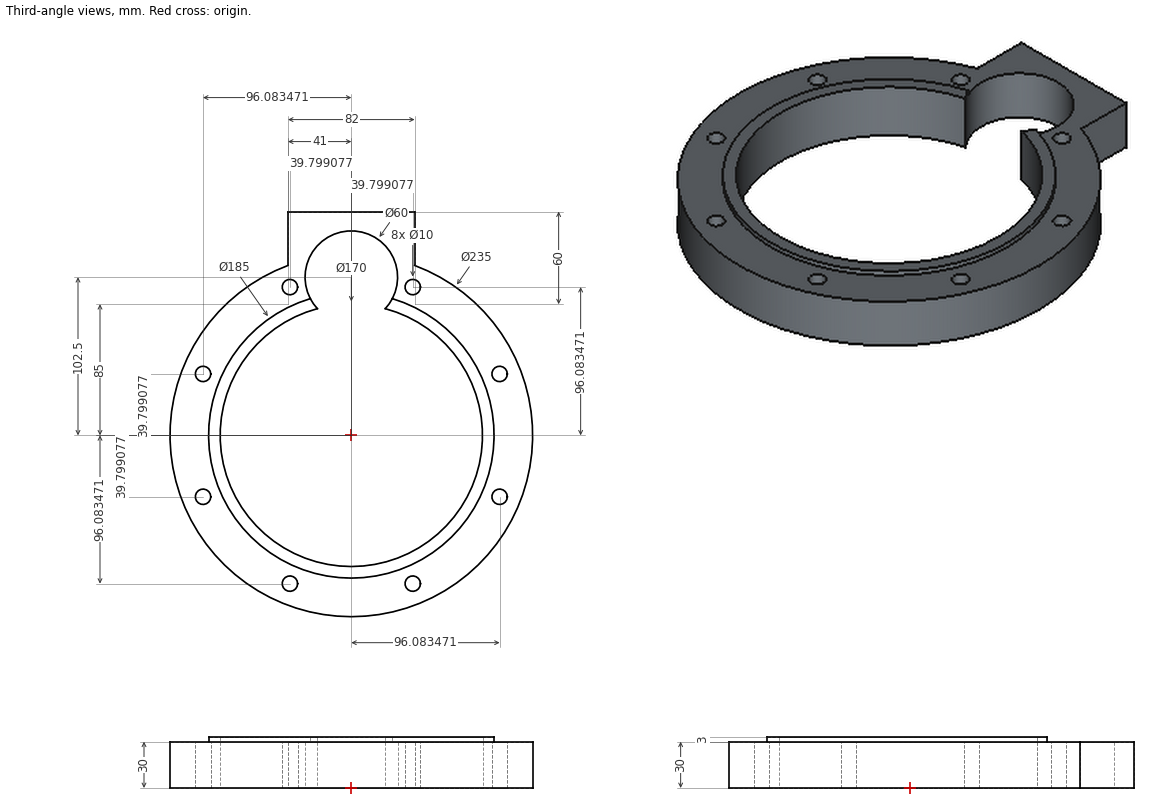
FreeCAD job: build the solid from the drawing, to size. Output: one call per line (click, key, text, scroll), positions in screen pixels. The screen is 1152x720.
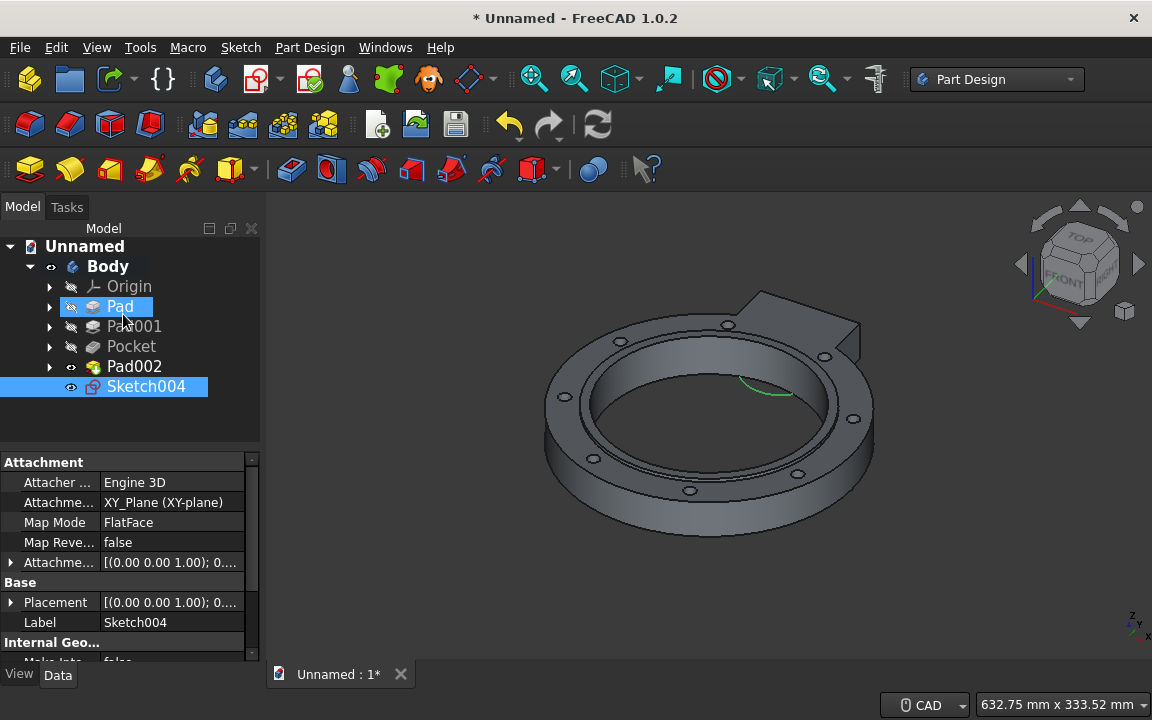
click(292, 170)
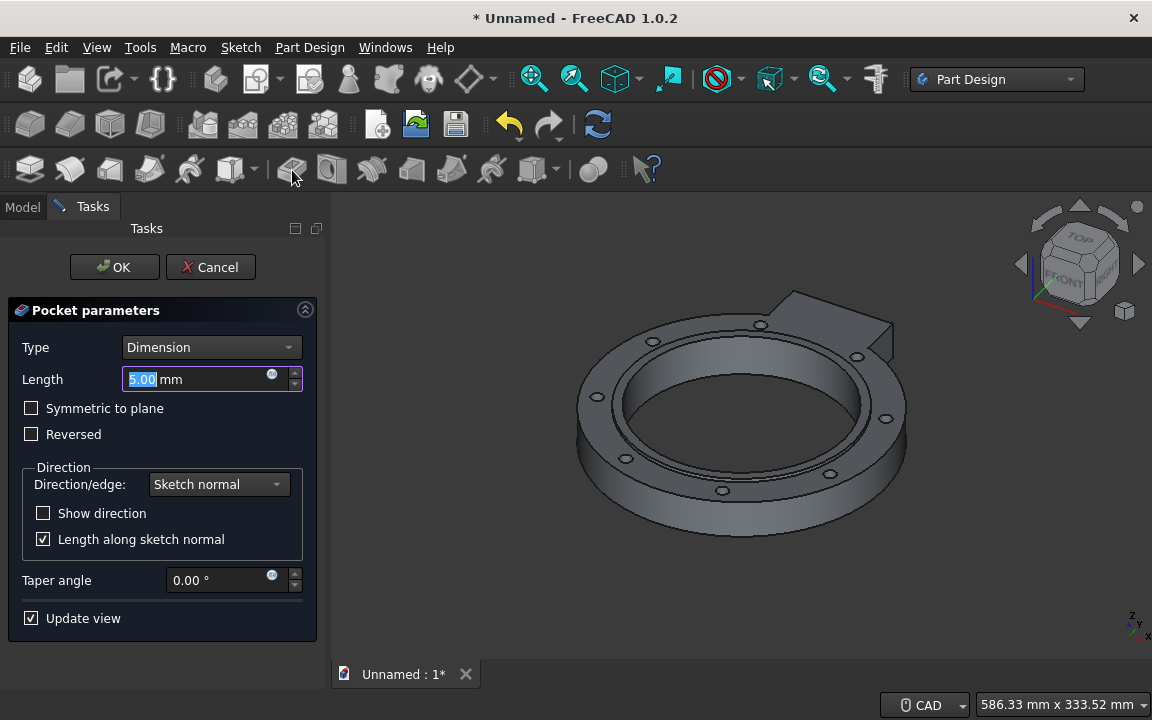
click(212, 348)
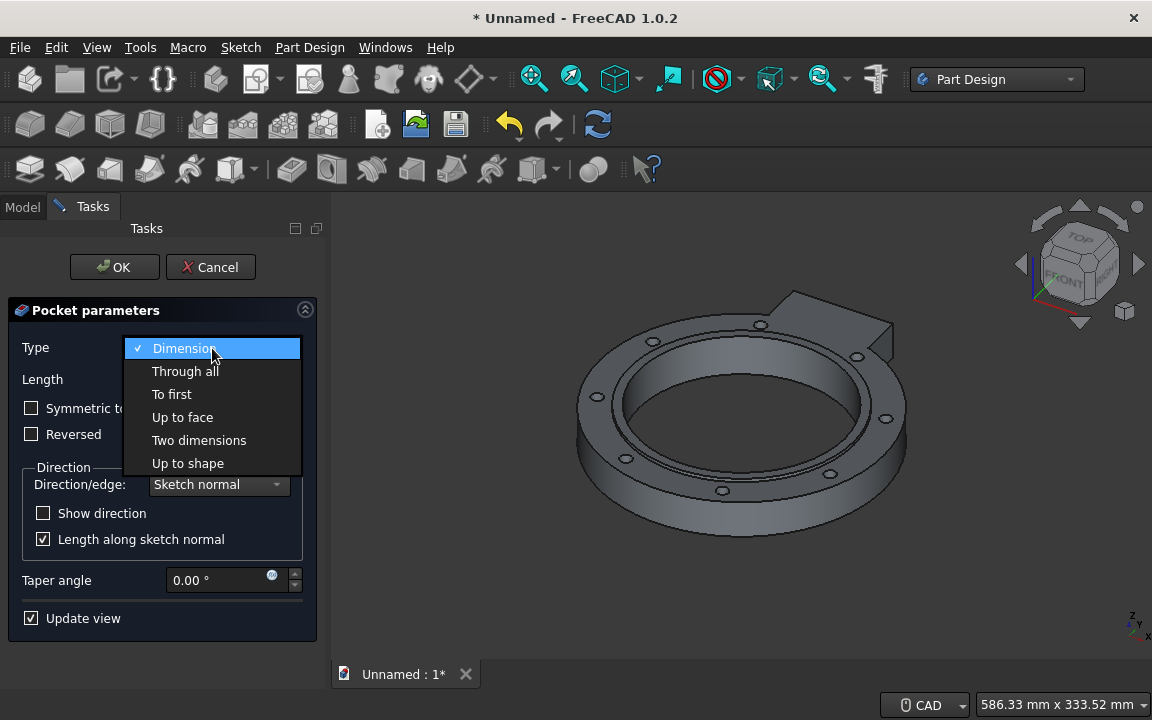
click(212, 372)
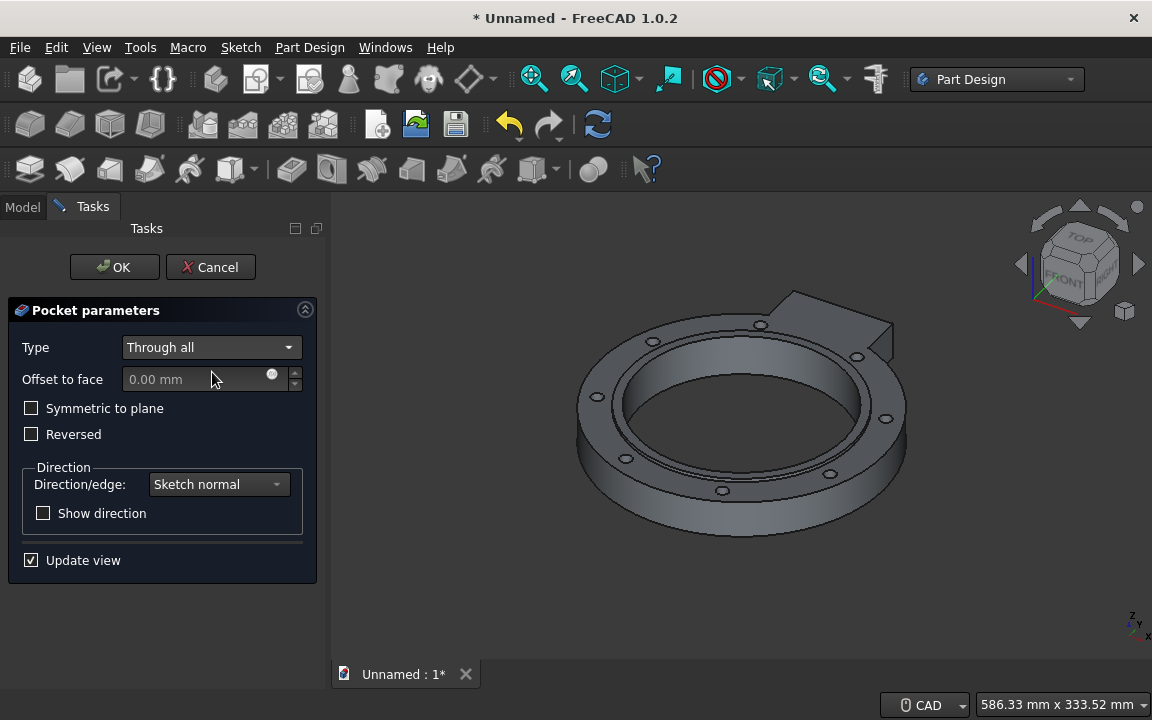
click(30, 434)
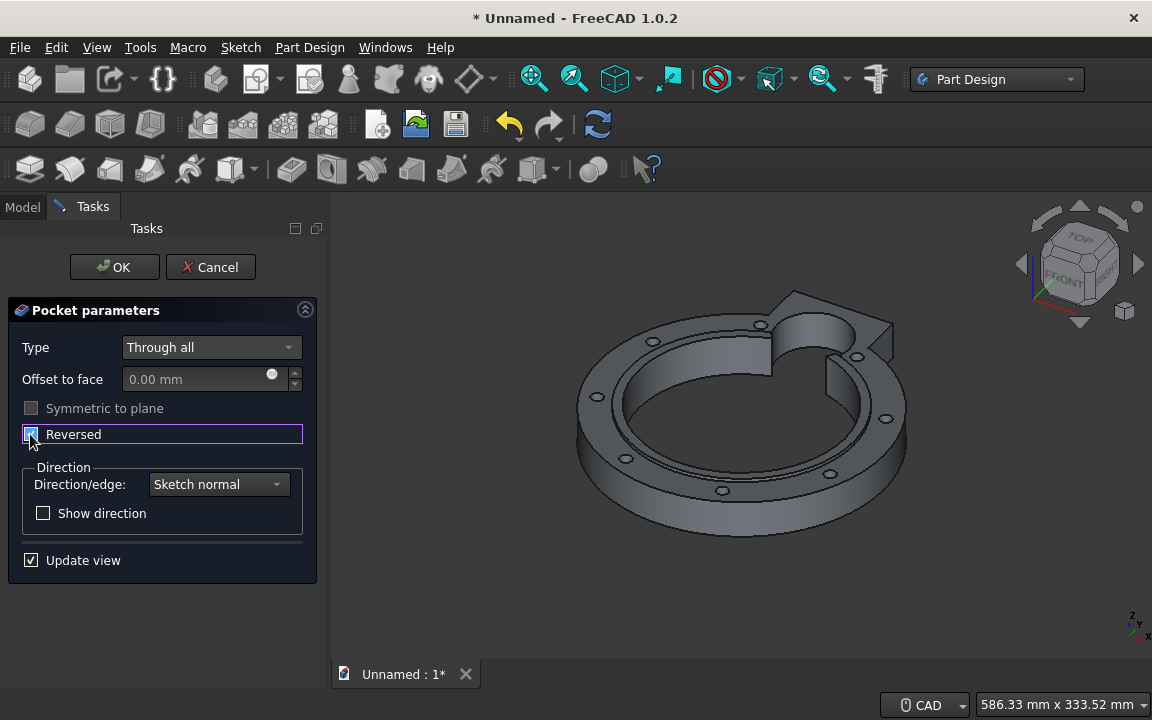
click(115, 267)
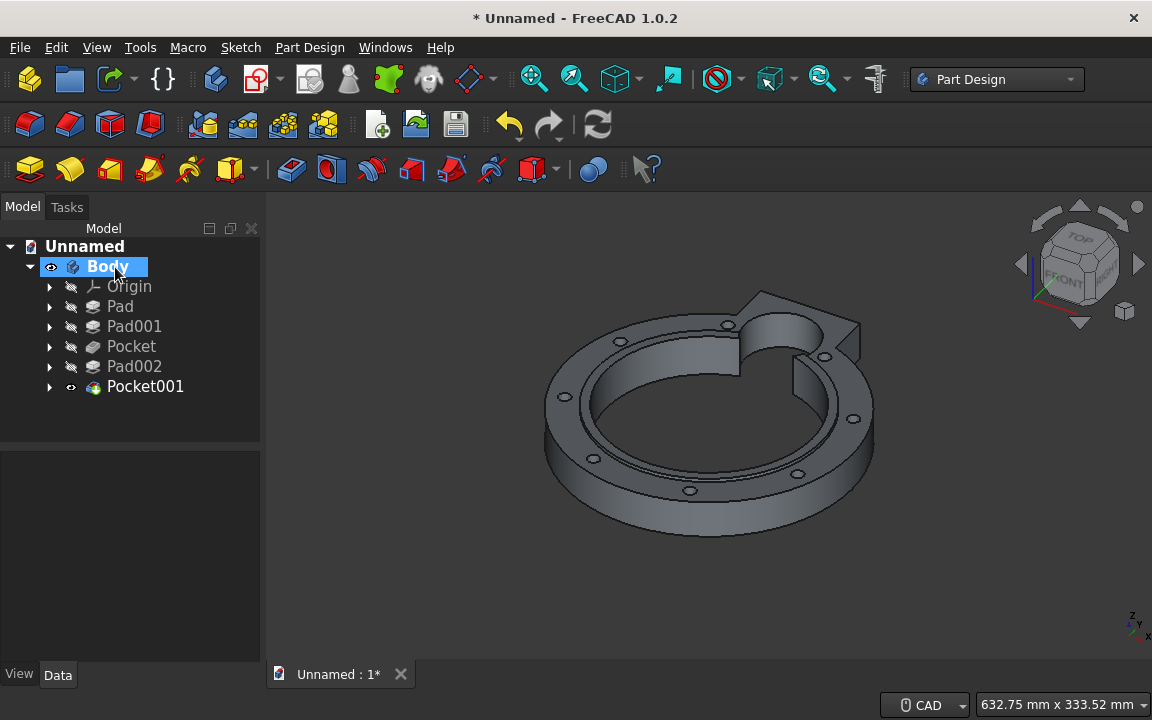
key(0)